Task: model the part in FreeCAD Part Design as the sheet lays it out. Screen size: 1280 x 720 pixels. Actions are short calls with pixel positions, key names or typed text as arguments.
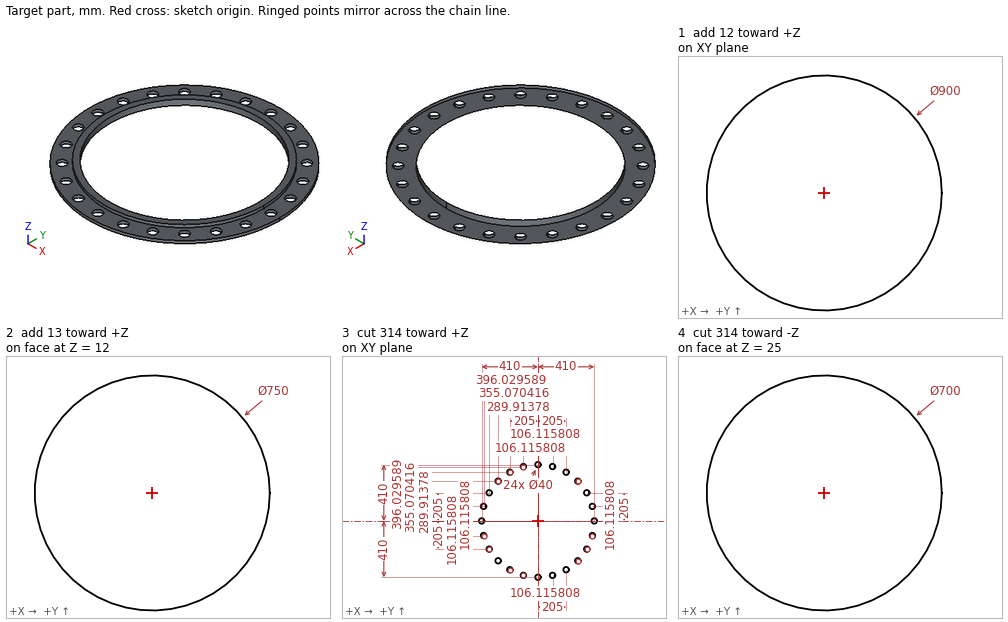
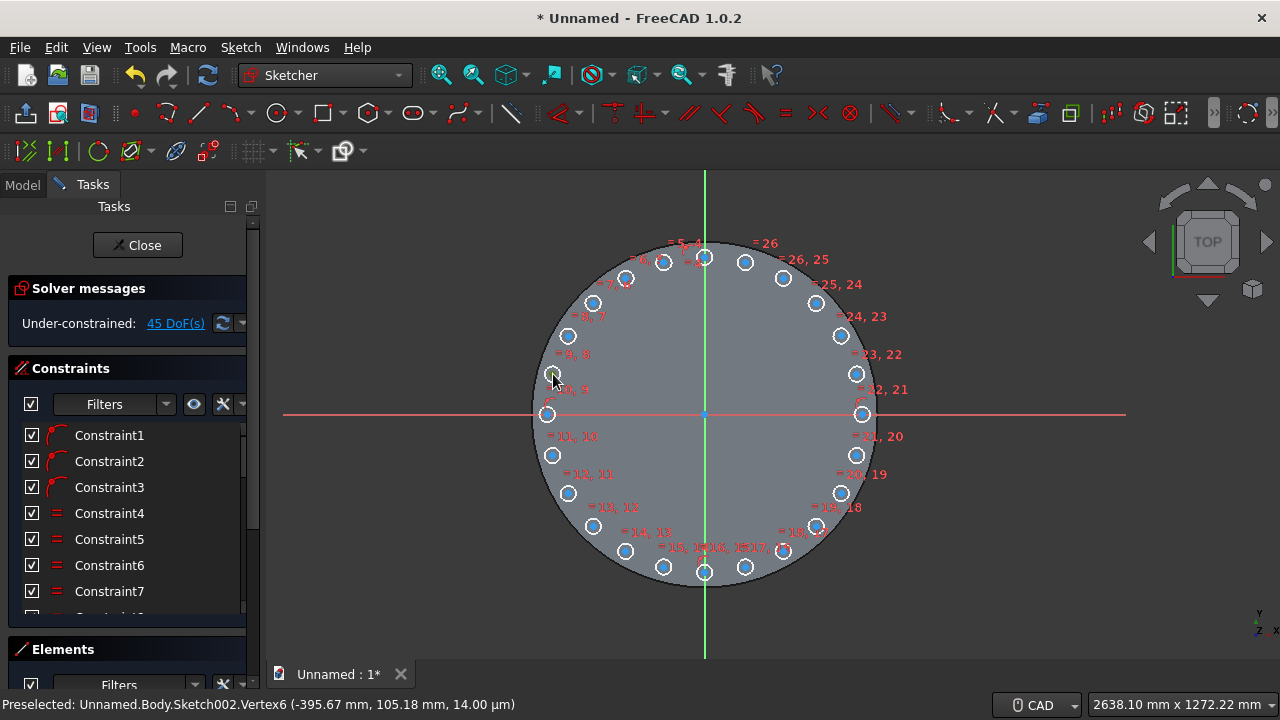
click(553, 456)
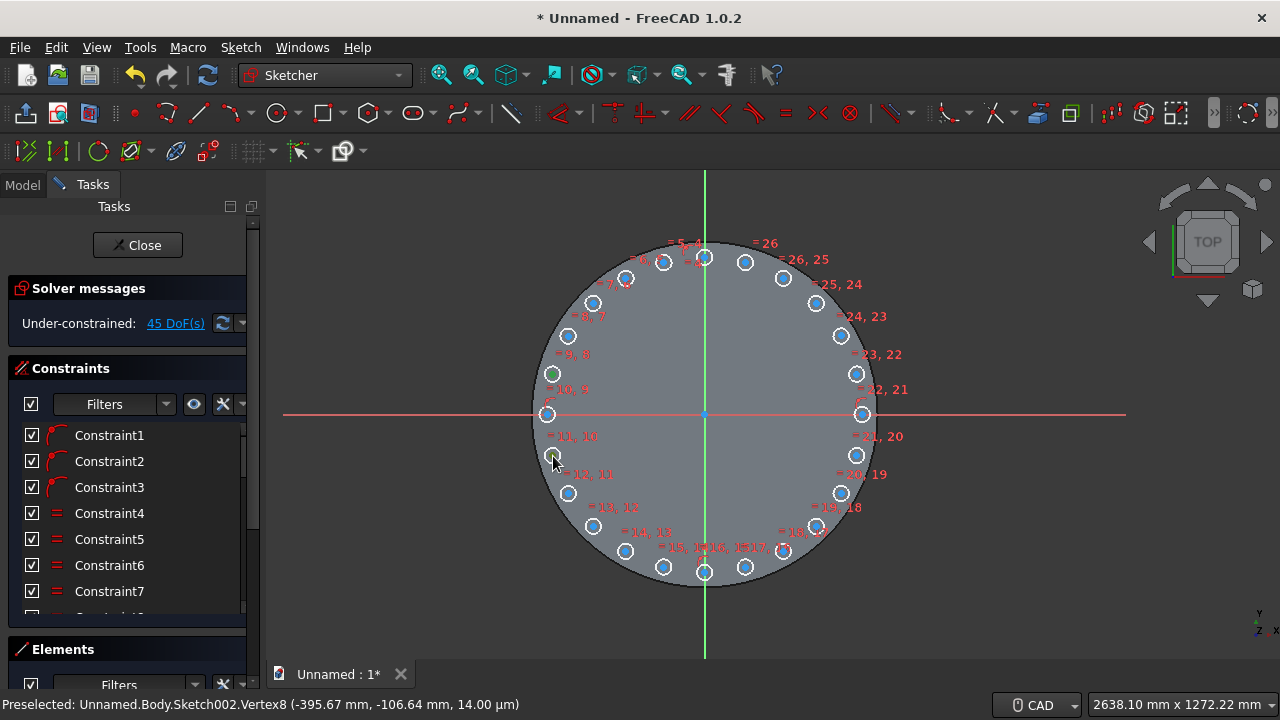
key(v)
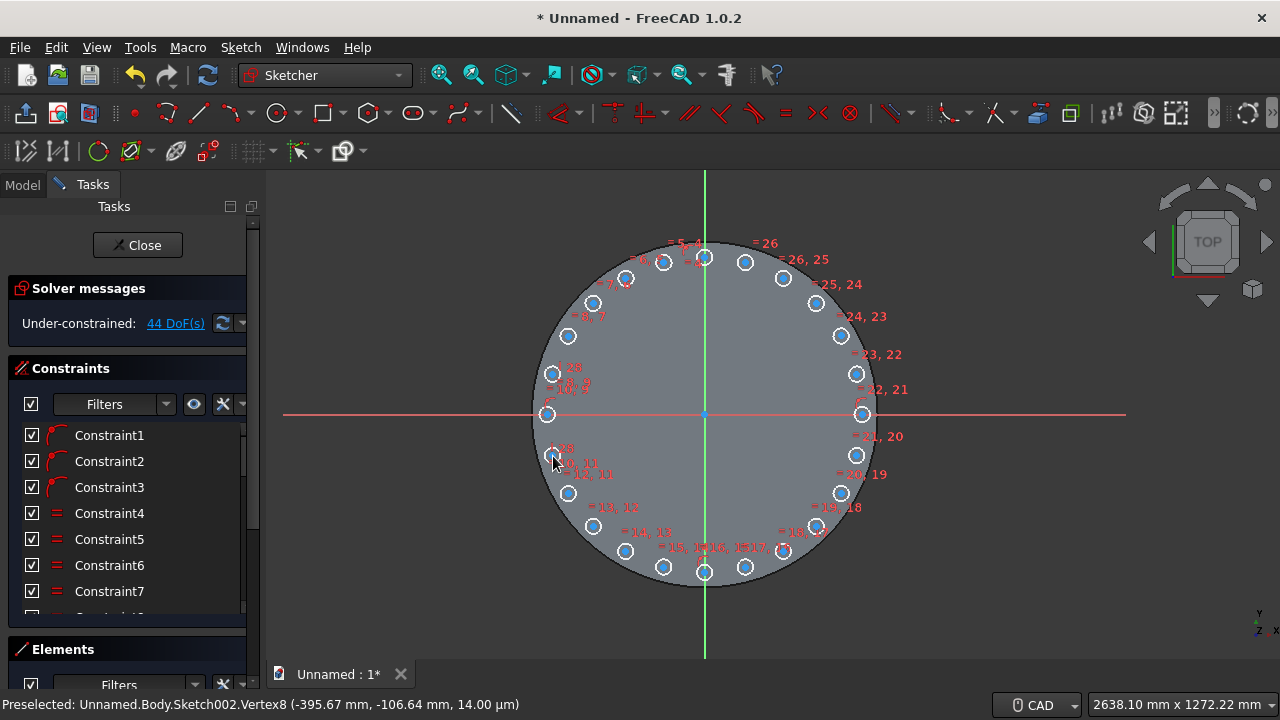
click(568, 336)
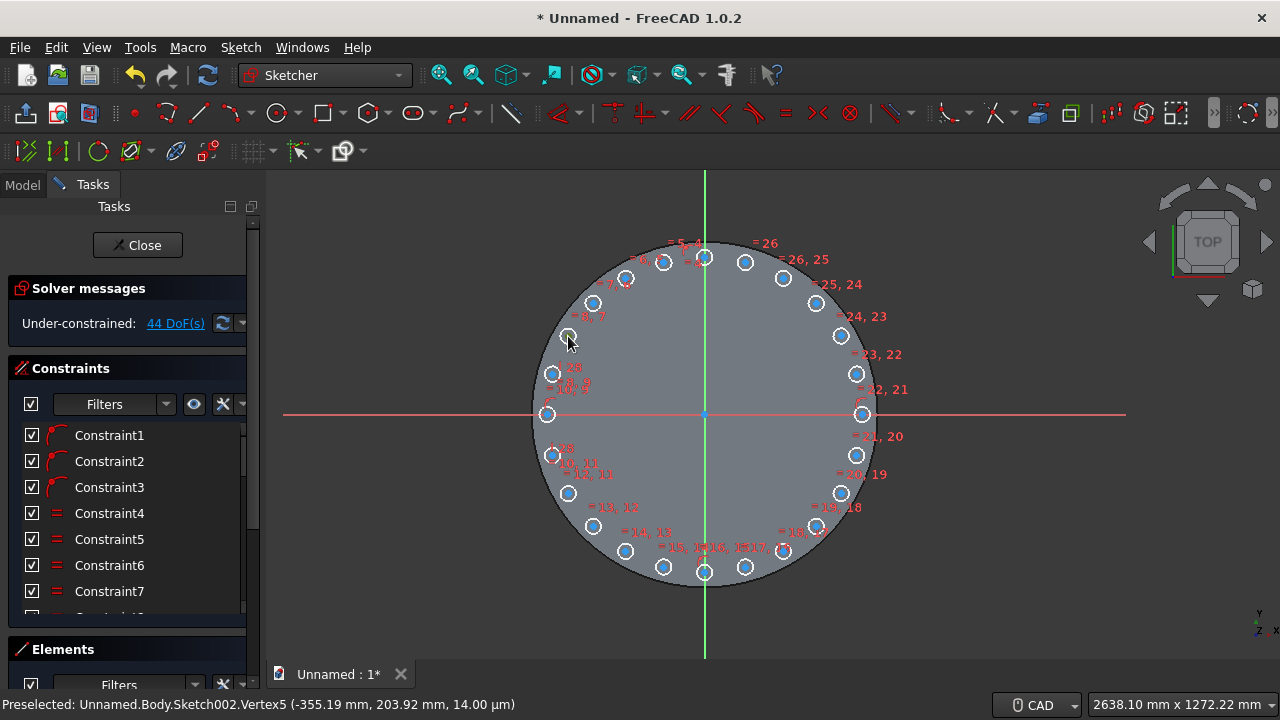
click(568, 494)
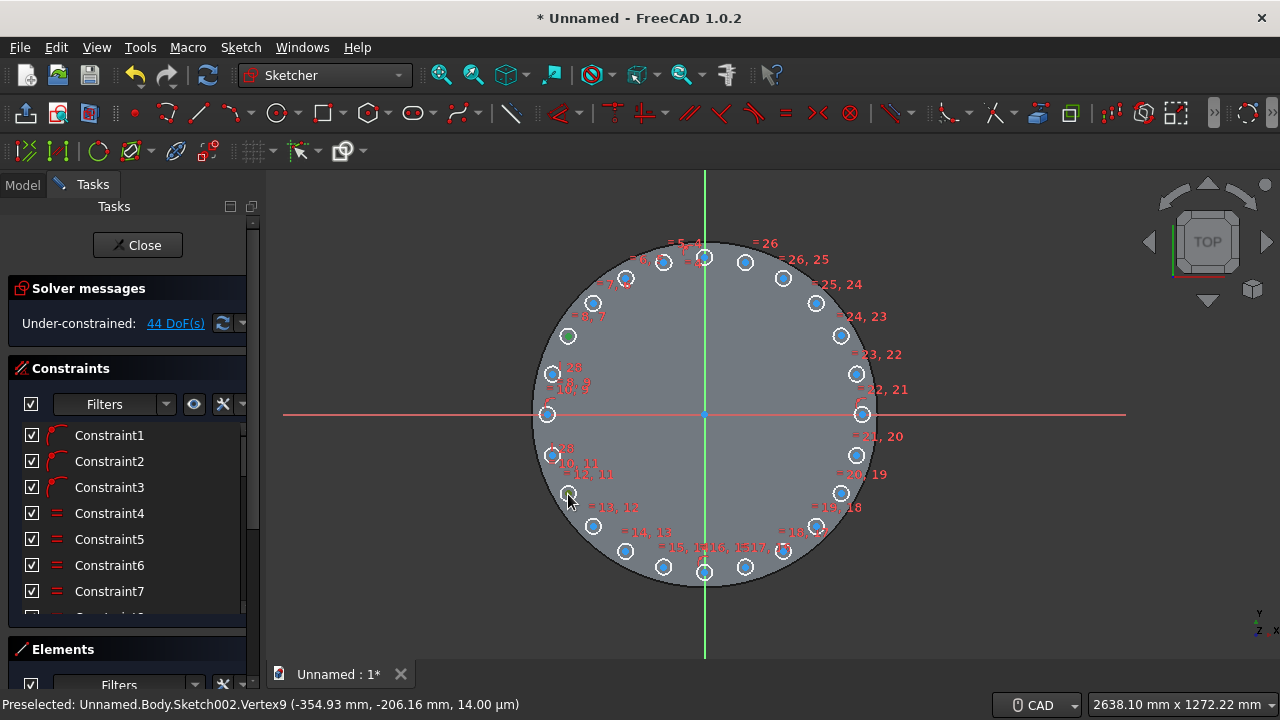
click(668, 114)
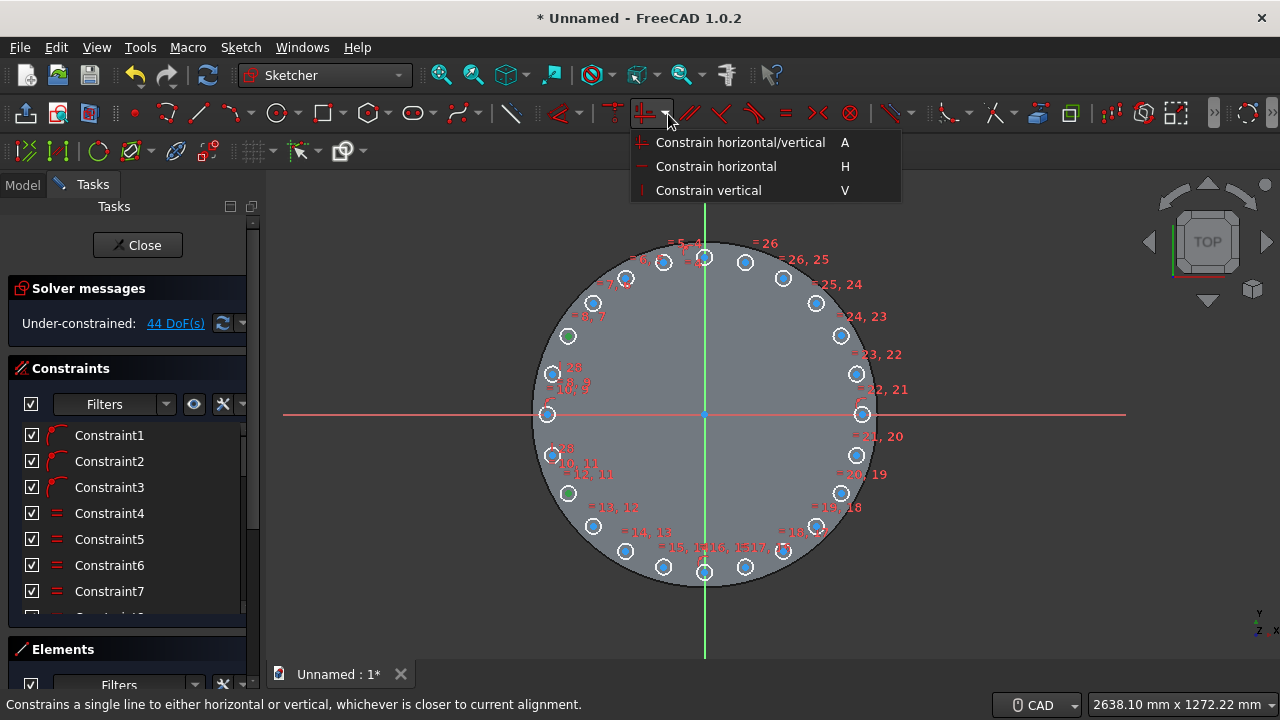
click(766, 190)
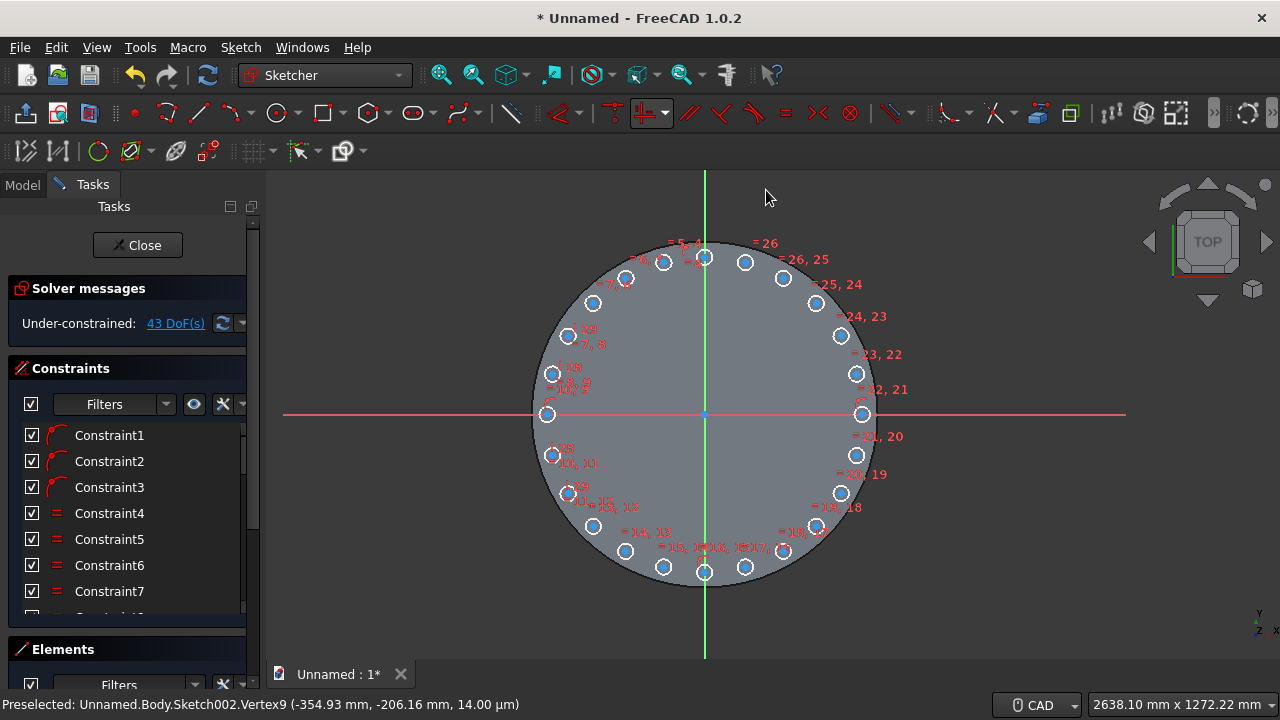
click(593, 303)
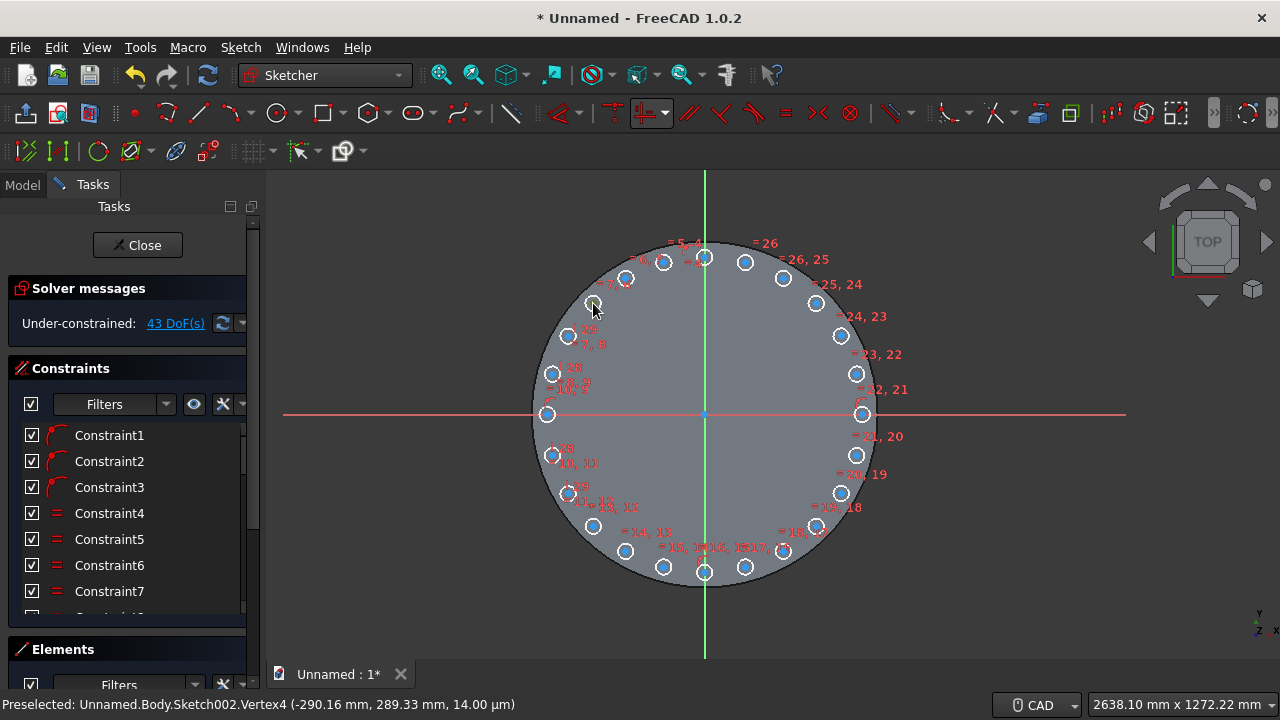
click(593, 526)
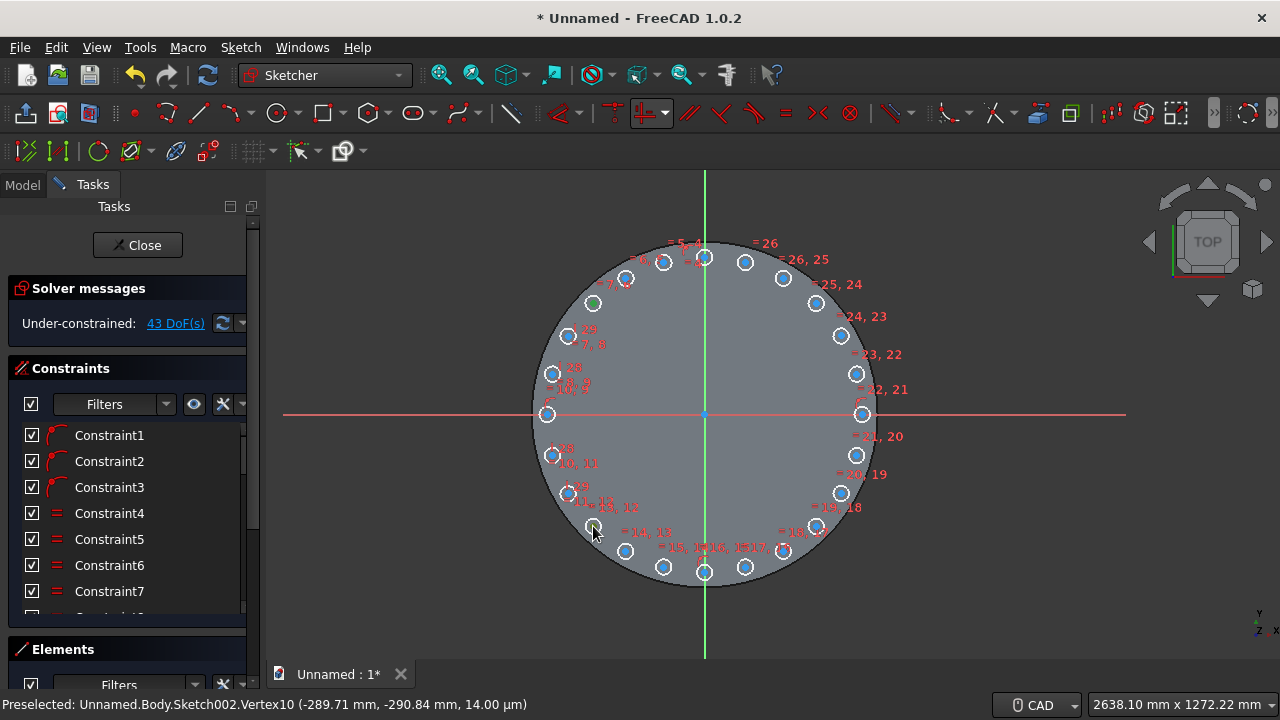
click(668, 114)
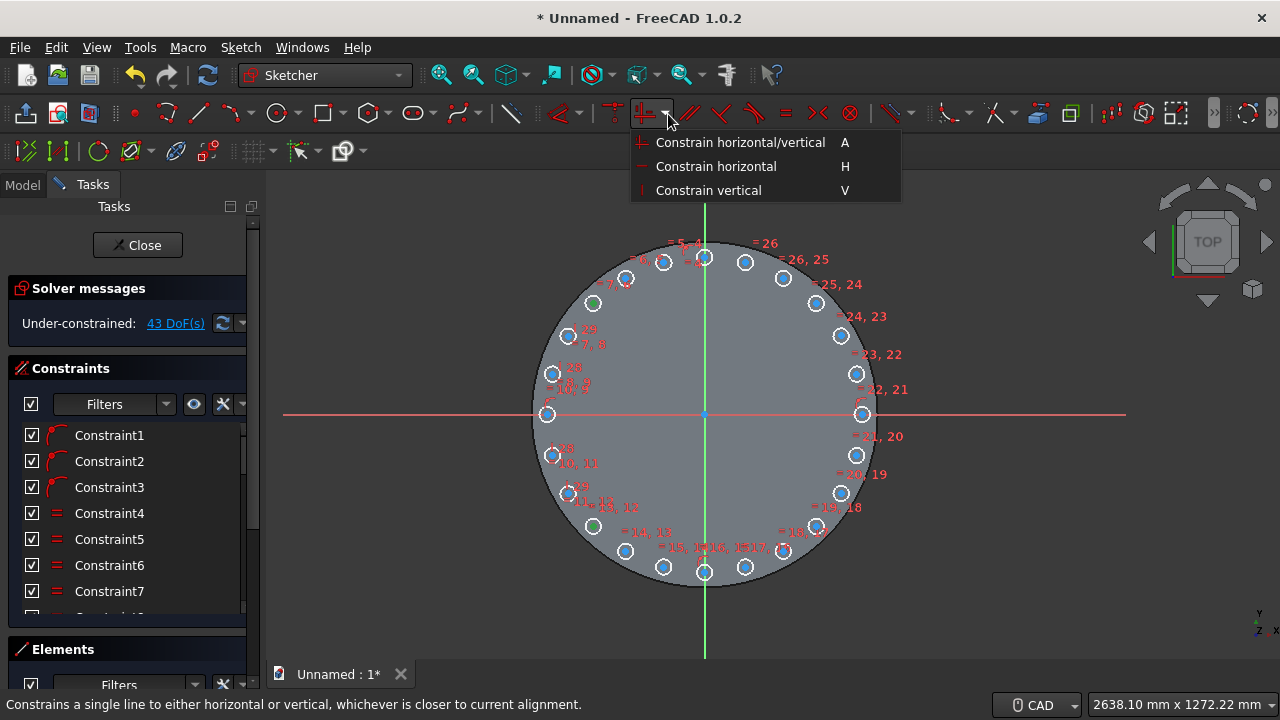
click(766, 190)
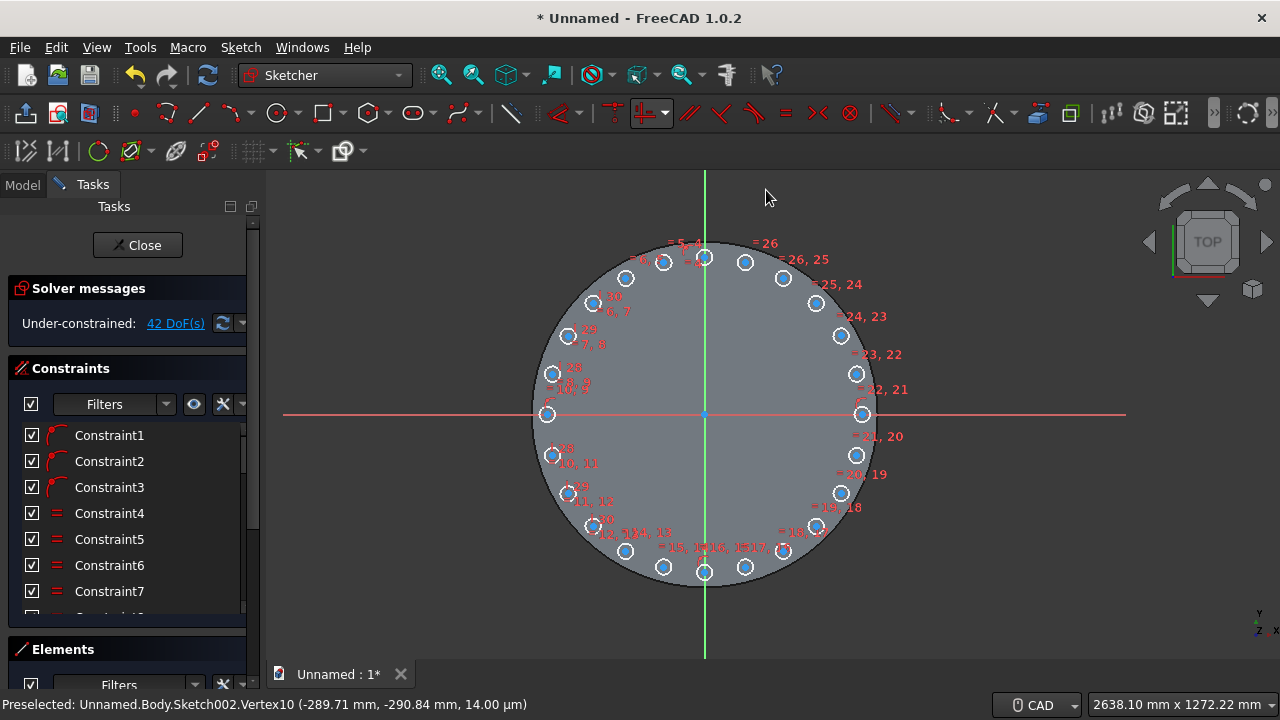
click(664, 567)